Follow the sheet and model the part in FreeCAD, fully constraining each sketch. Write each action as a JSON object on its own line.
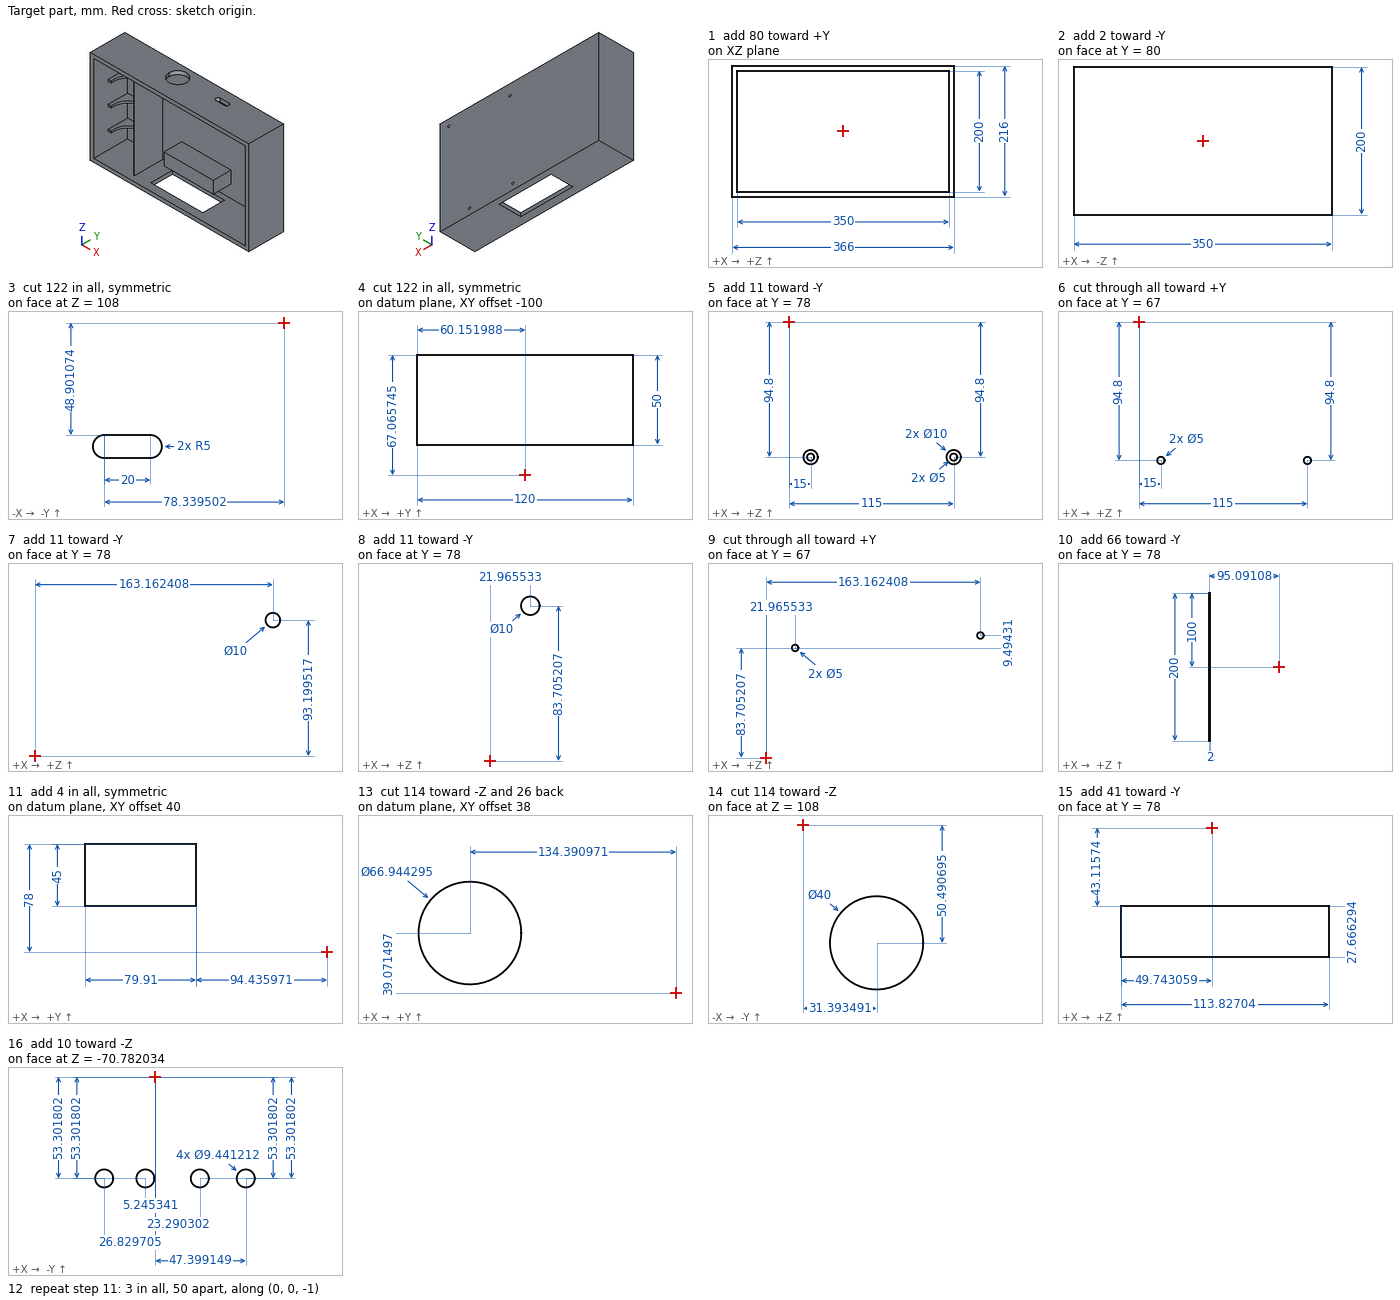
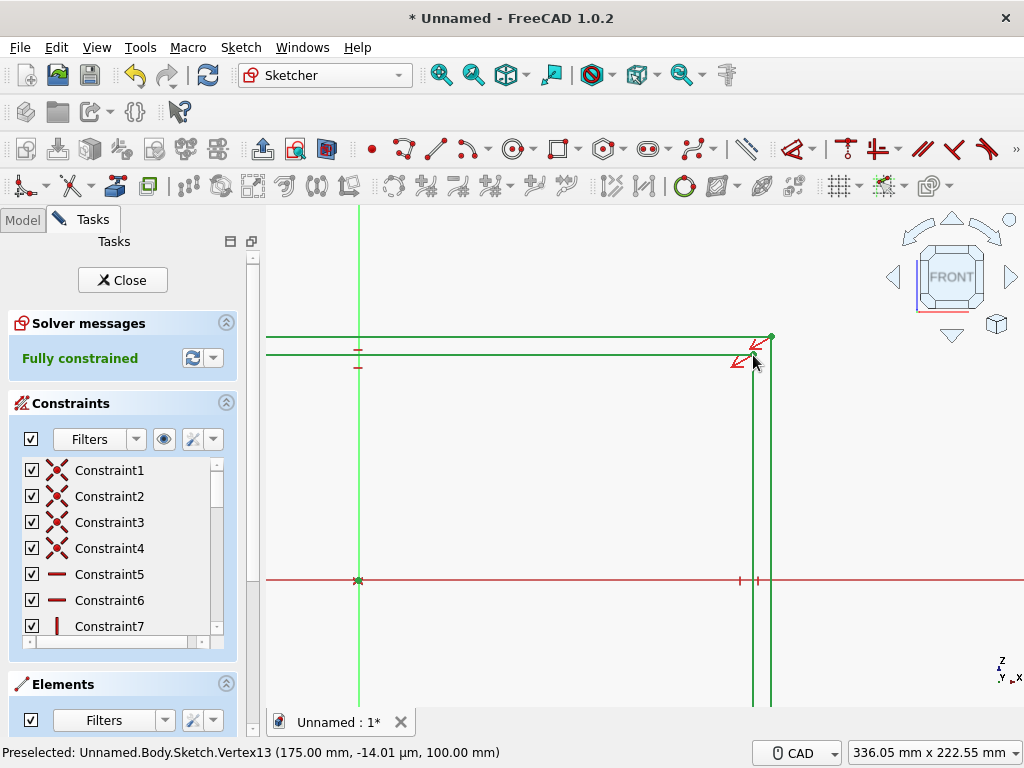
{"action": "left_click", "coordinate": [123, 280]}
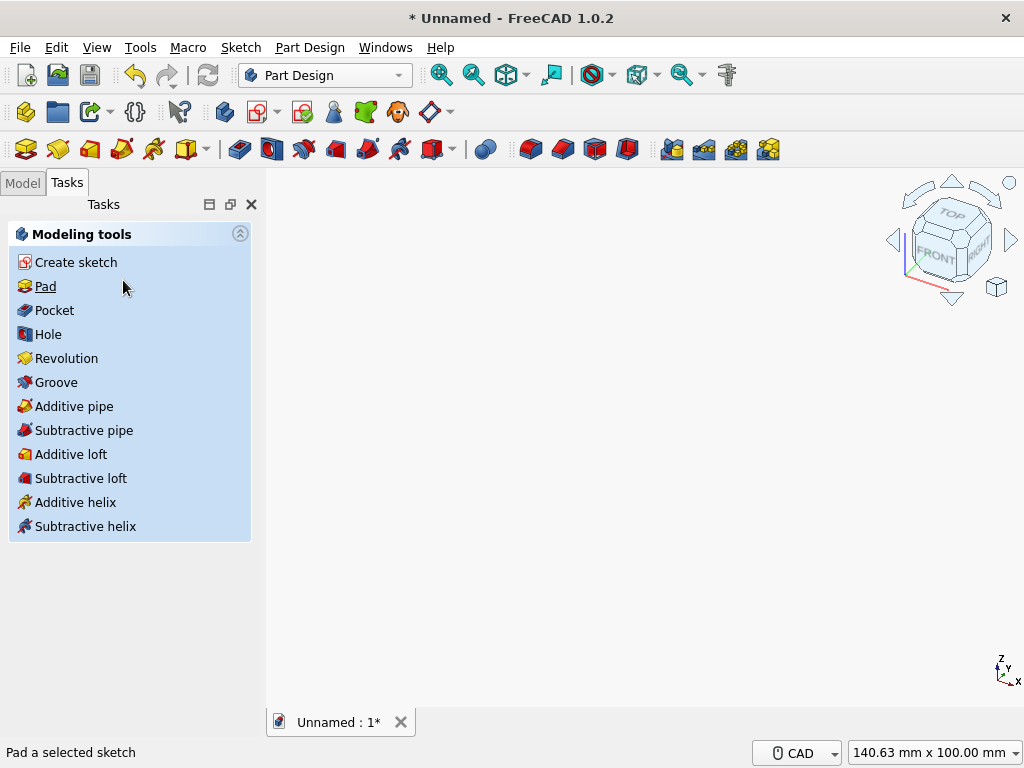
{"action": "left_click", "coordinate": [26, 150]}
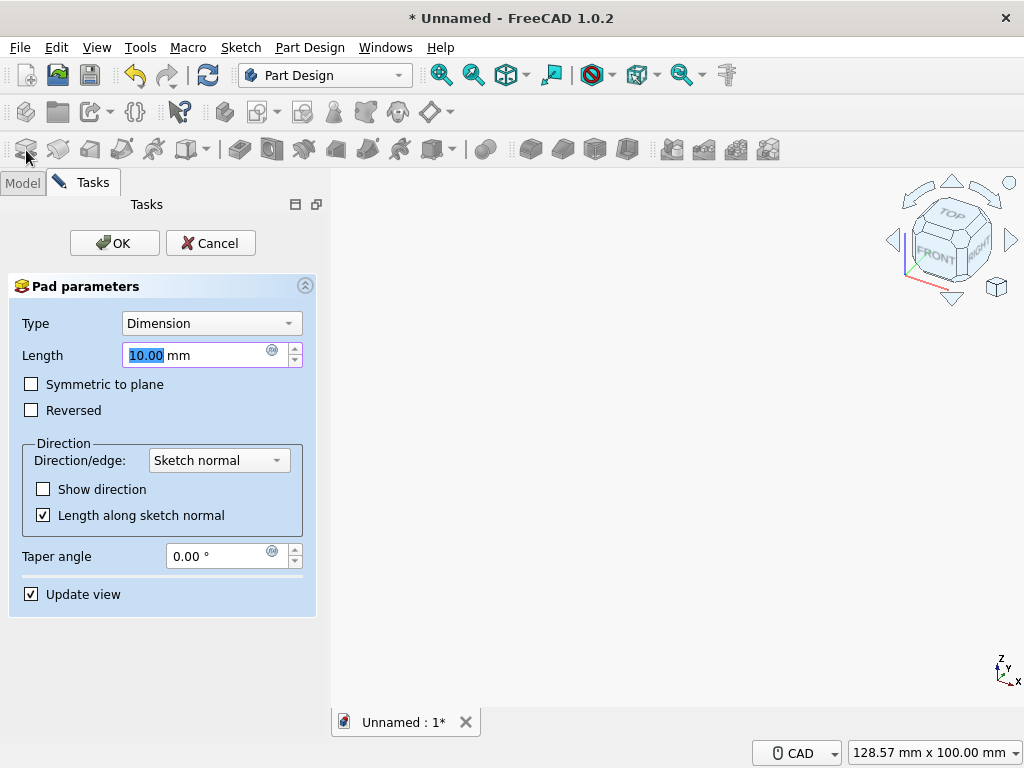
{"action": "type", "text": "80"}
{"action": "key", "text": "Tab"}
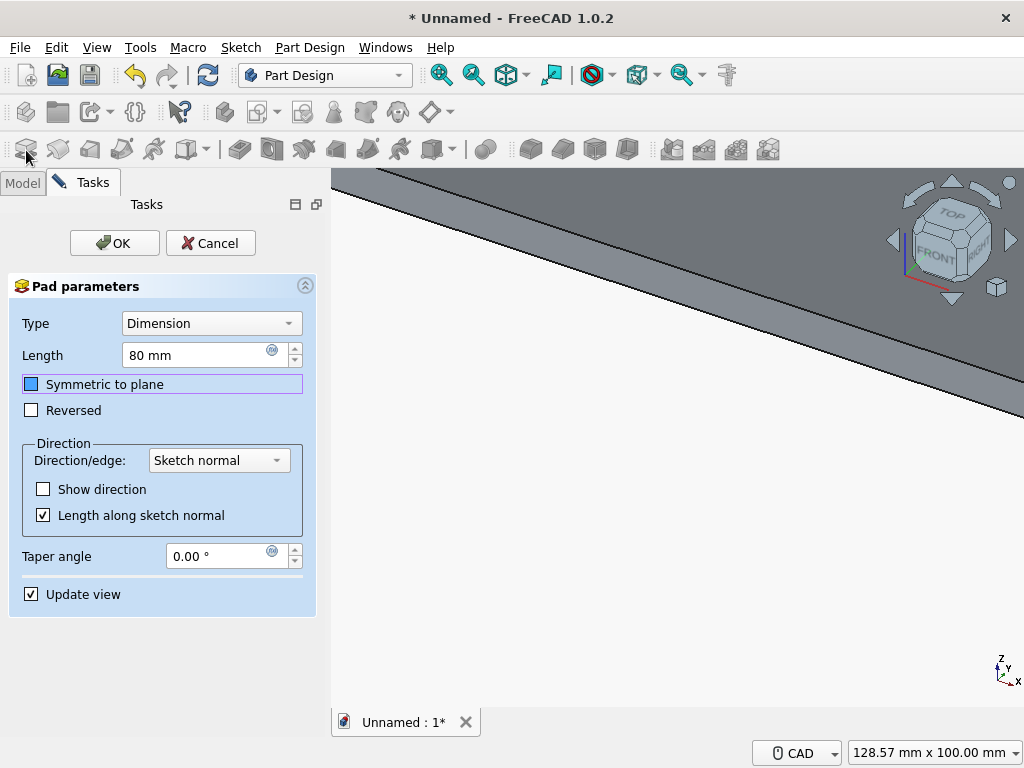
{"action": "left_click", "coordinate": [30, 410]}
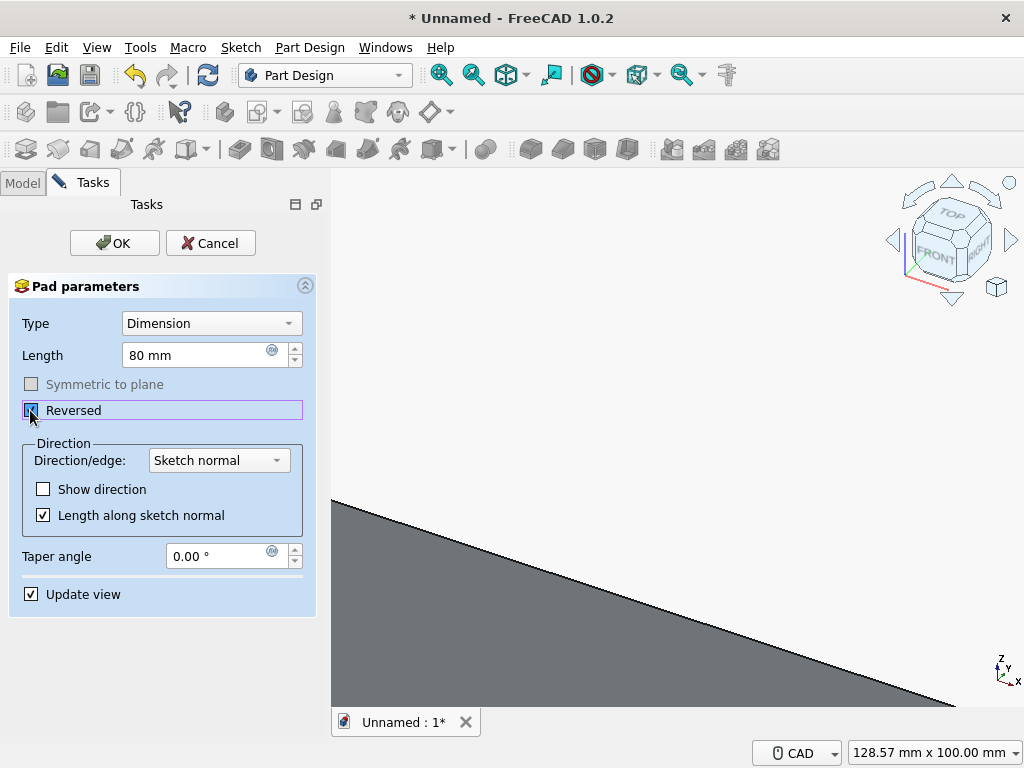
{"action": "left_click", "coordinate": [115, 243]}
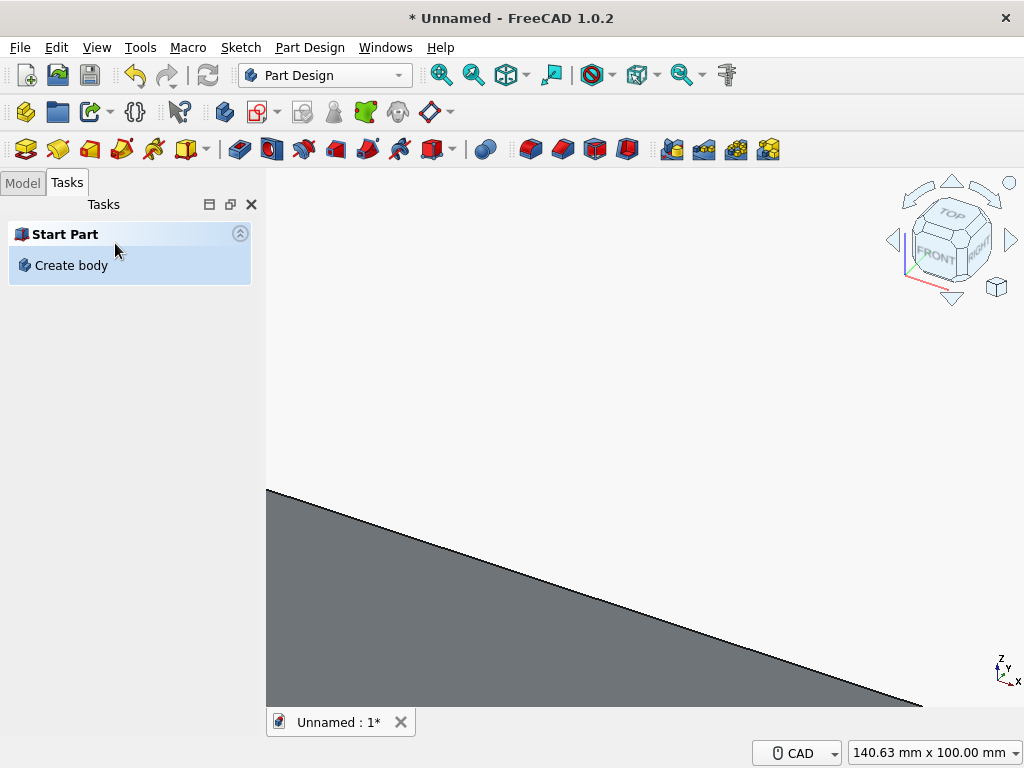
{"action": "left_click", "coordinate": [442, 76]}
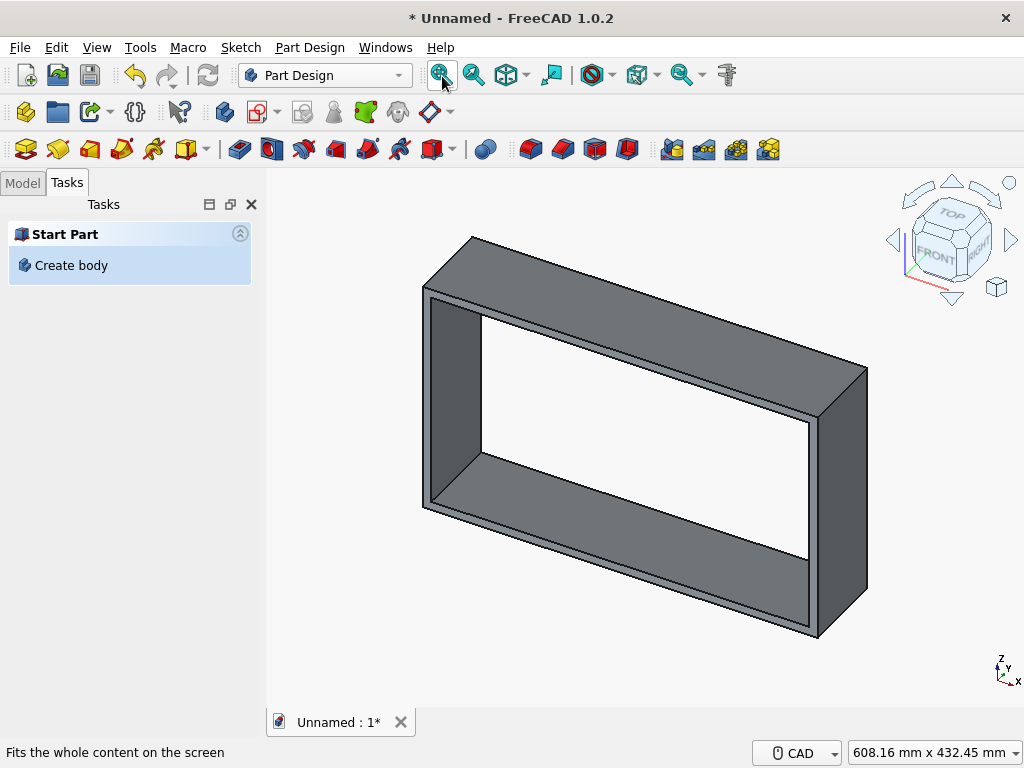
{"action": "key", "text": "4"}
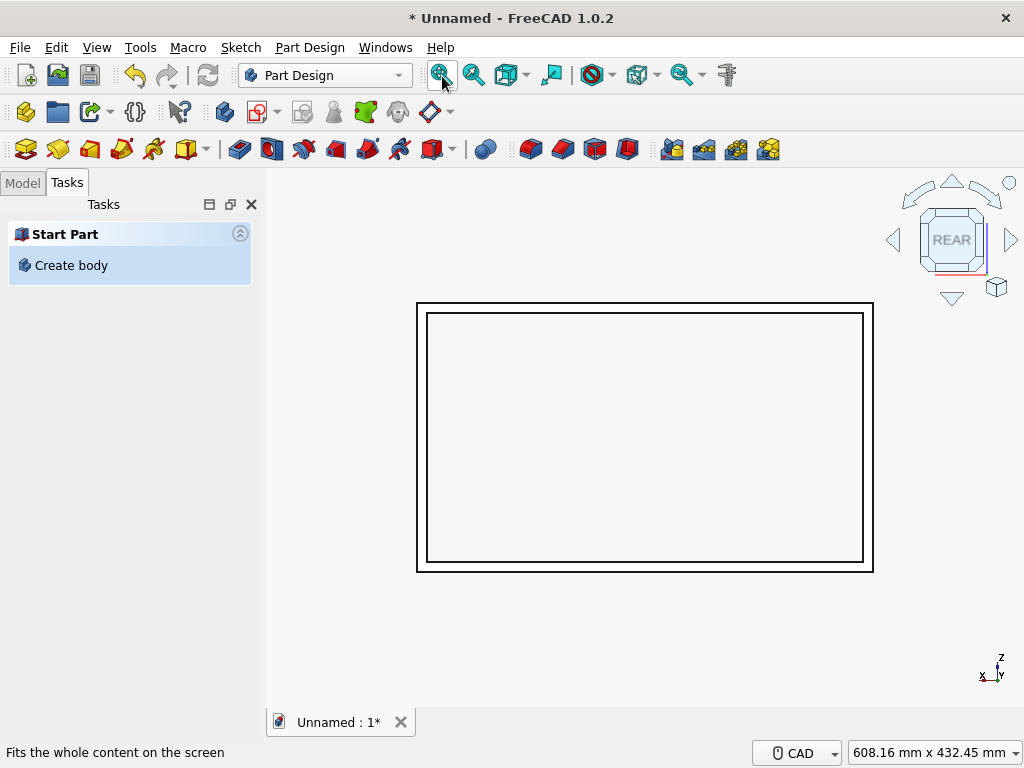
{"action": "scroll", "coordinate": [424, 481], "scroll_direction": "up", "scroll_amount": 7}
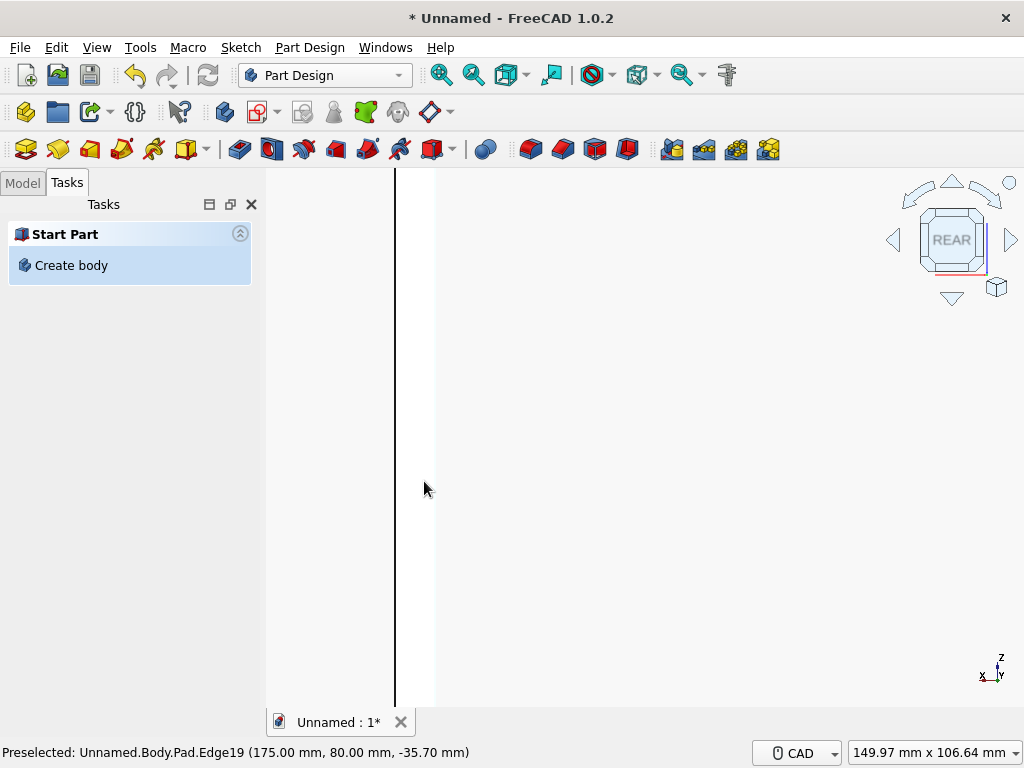
{"action": "left_click", "coordinate": [422, 484]}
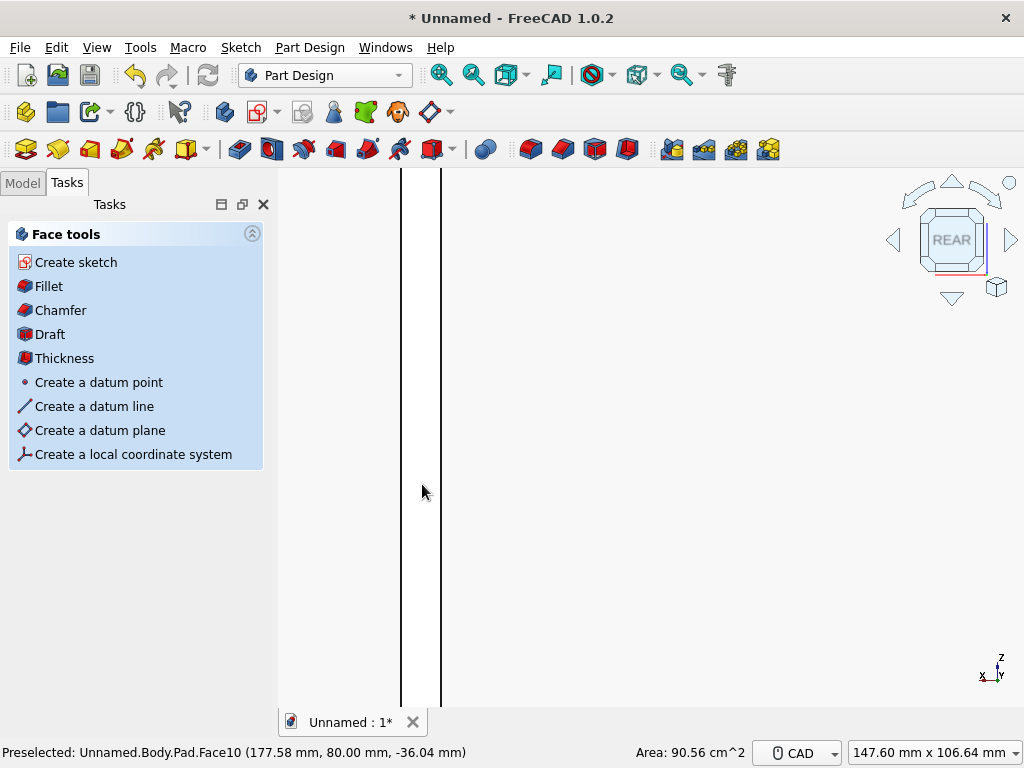
{"action": "left_click", "coordinate": [258, 112]}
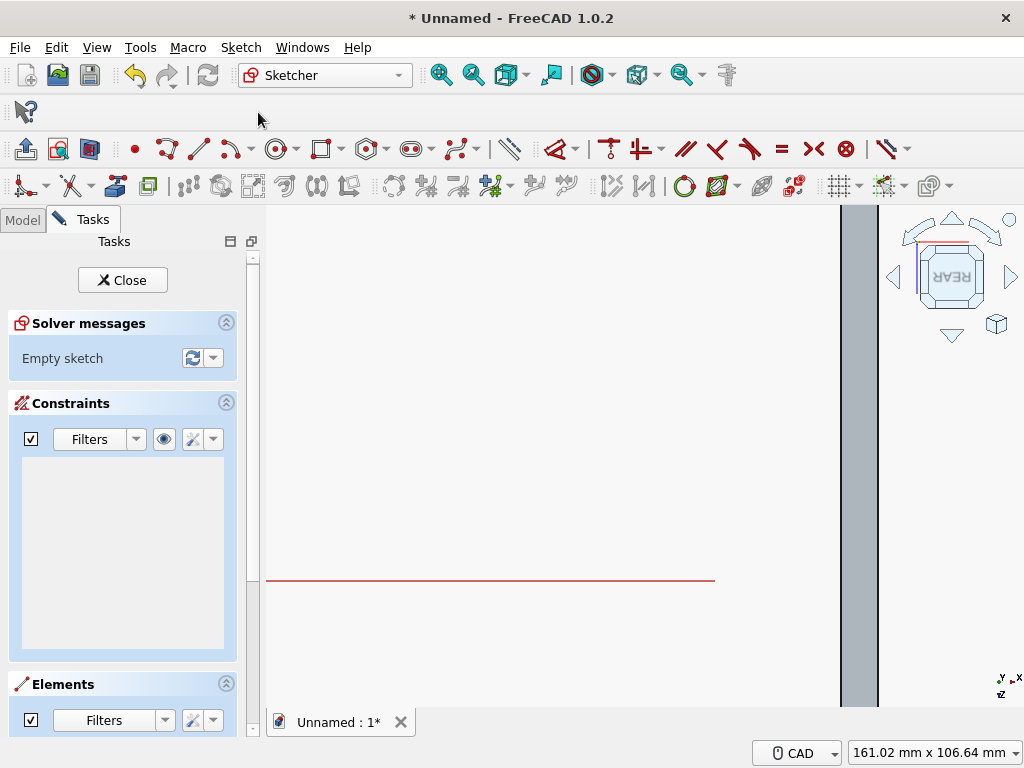
{"action": "scroll", "coordinate": [760, 415], "scroll_direction": "down", "scroll_amount": 7}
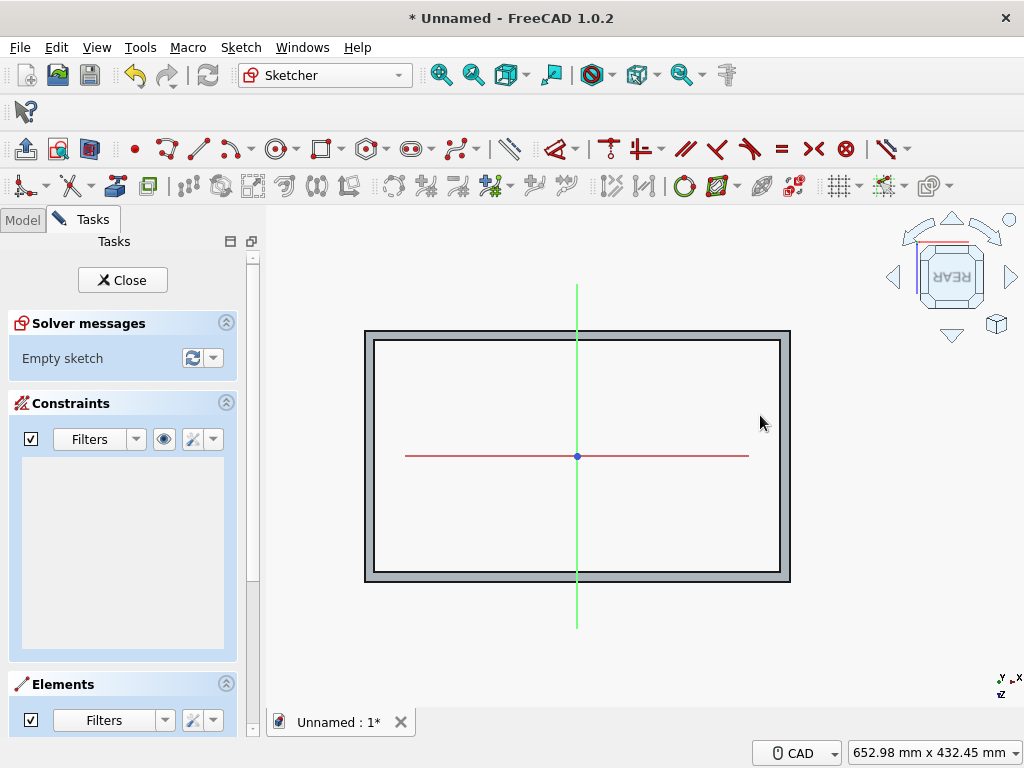
{"action": "key", "text": "g v"}